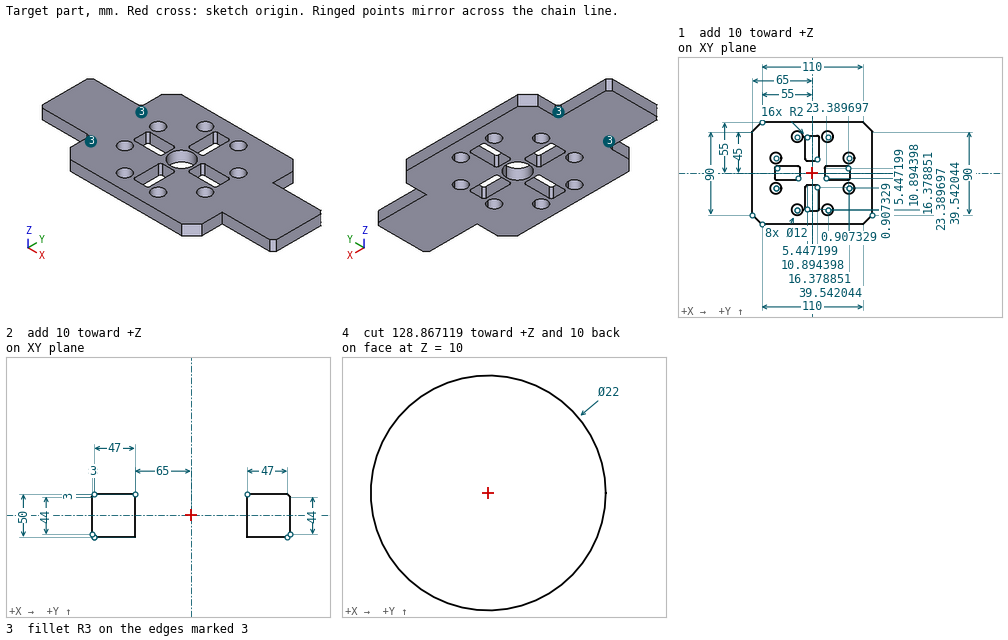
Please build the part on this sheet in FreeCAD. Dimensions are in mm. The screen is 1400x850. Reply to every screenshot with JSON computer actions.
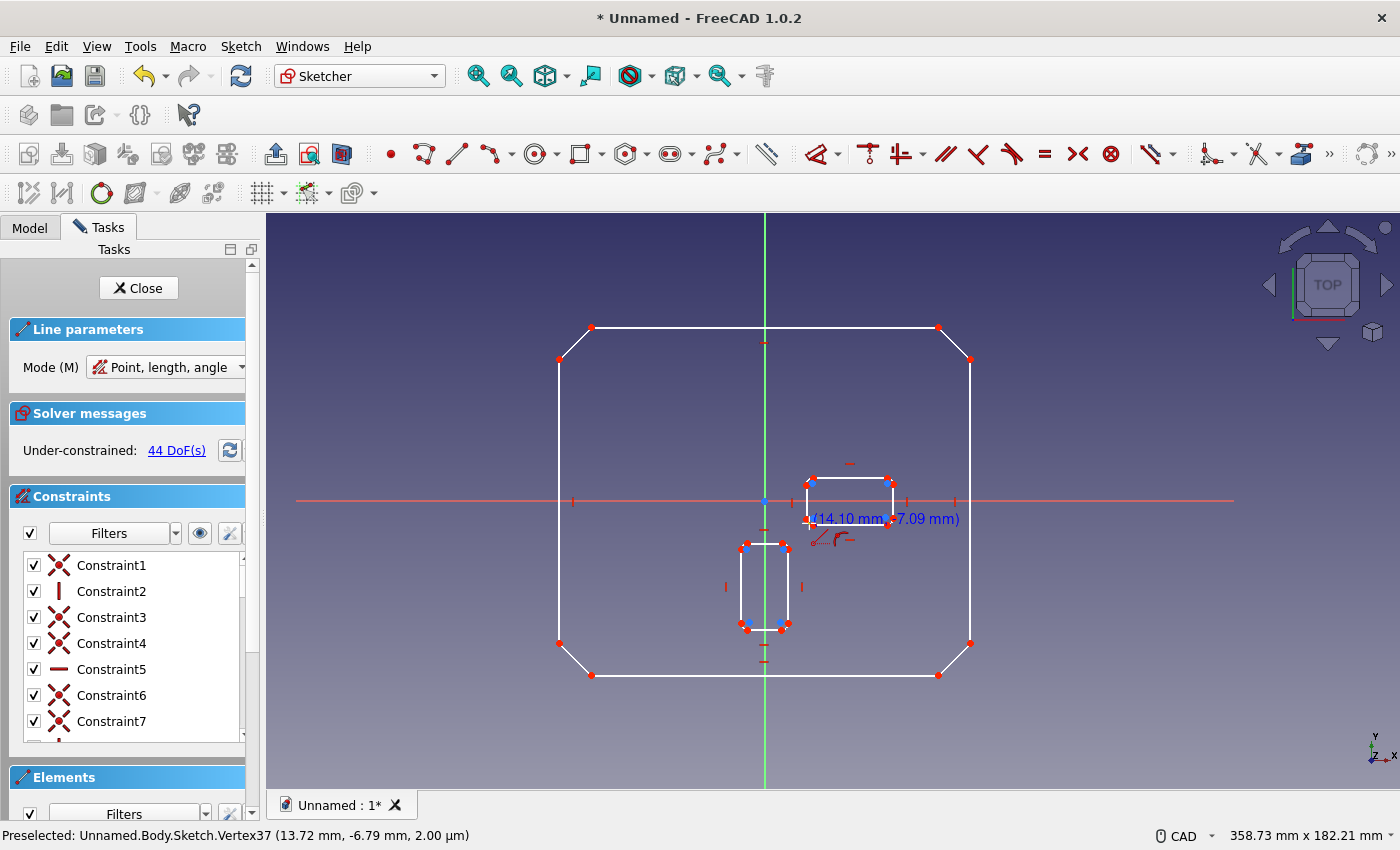
{"action": "left_click", "coordinate": [723, 484]}
{"action": "left_click", "coordinate": [723, 518]}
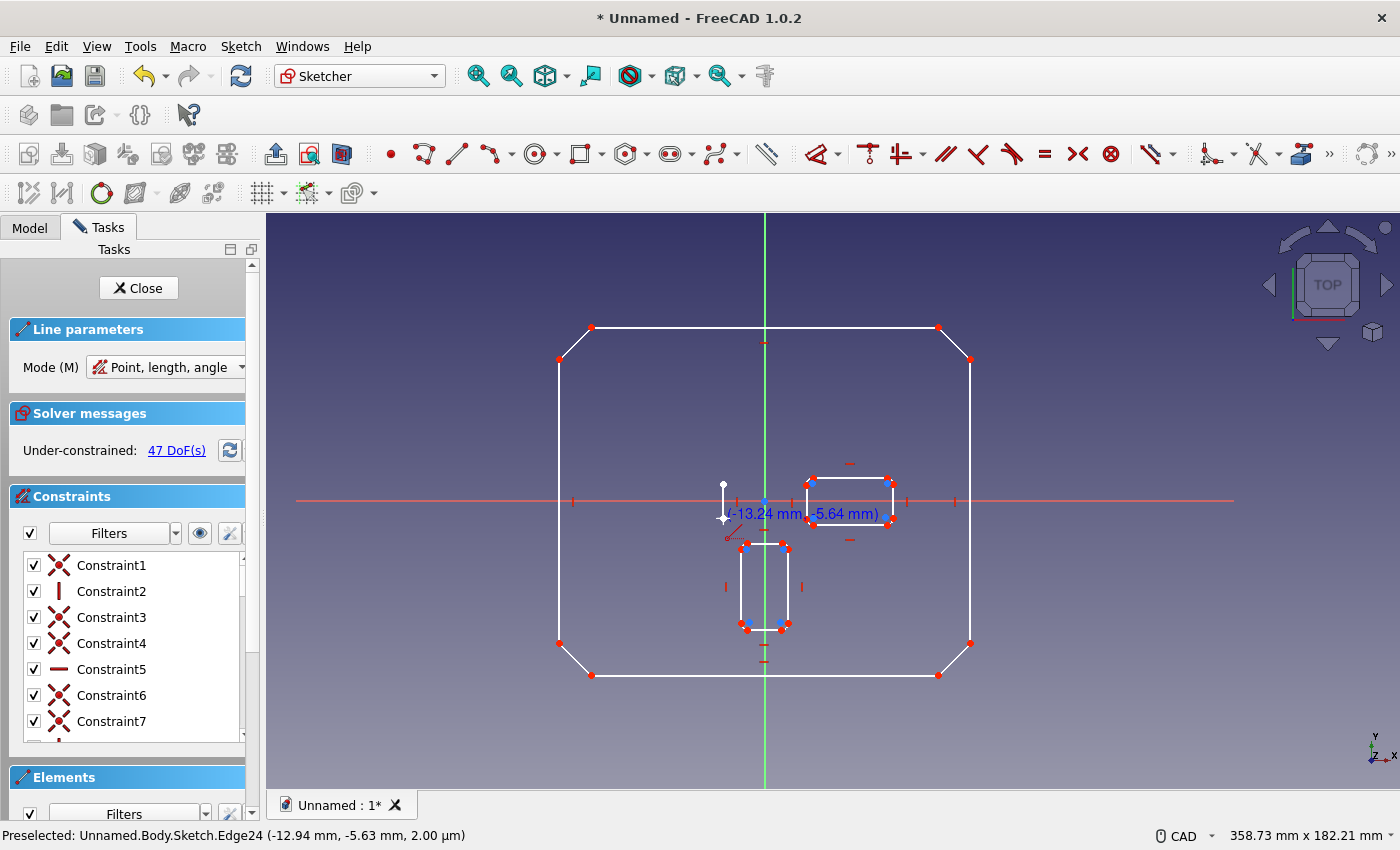
{"action": "scroll", "coordinate": [717, 525], "scroll_direction": "up", "scroll_amount": 3}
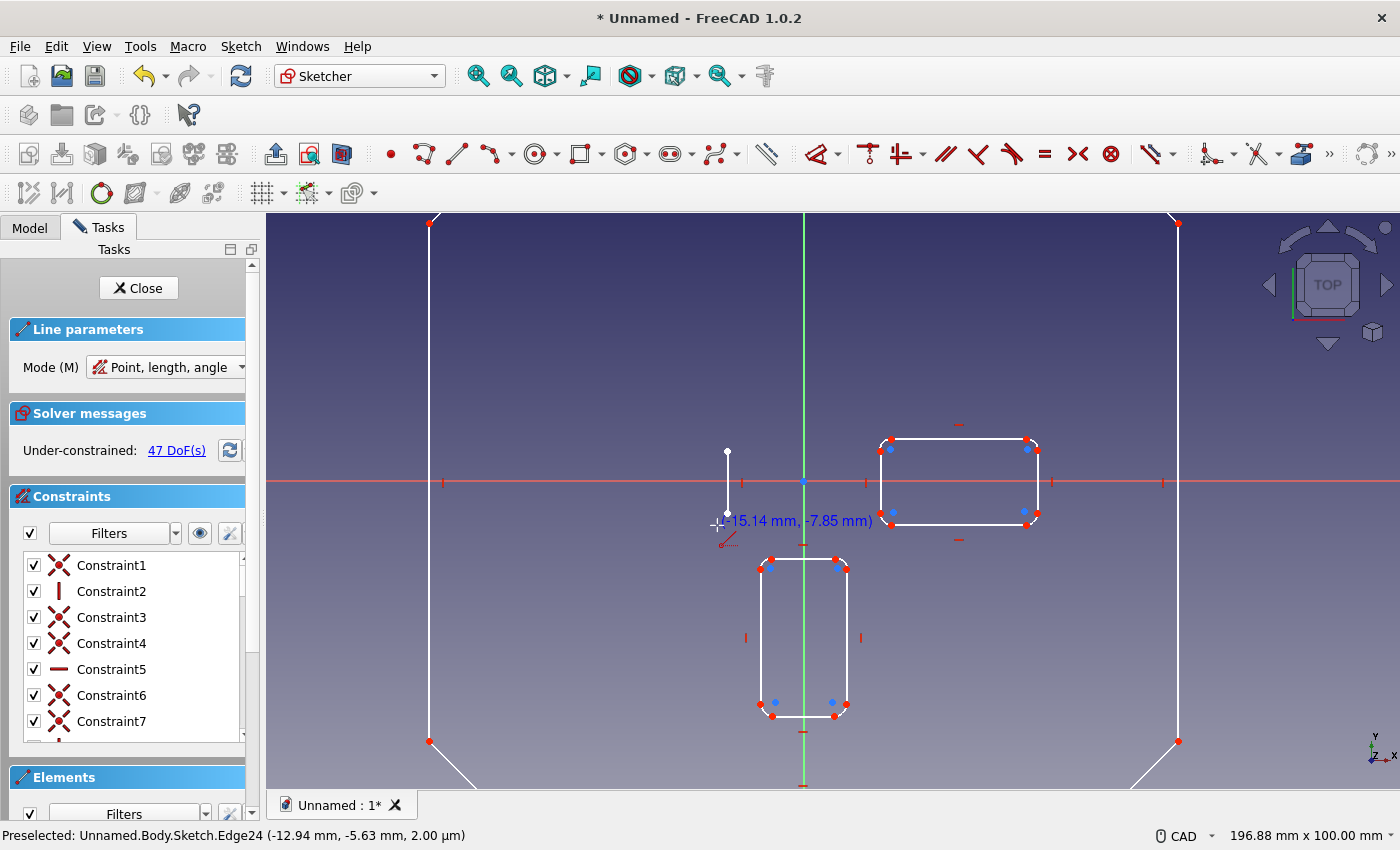
{"action": "left_click", "coordinate": [716, 524]}
{"action": "left_click", "coordinate": [581, 524]}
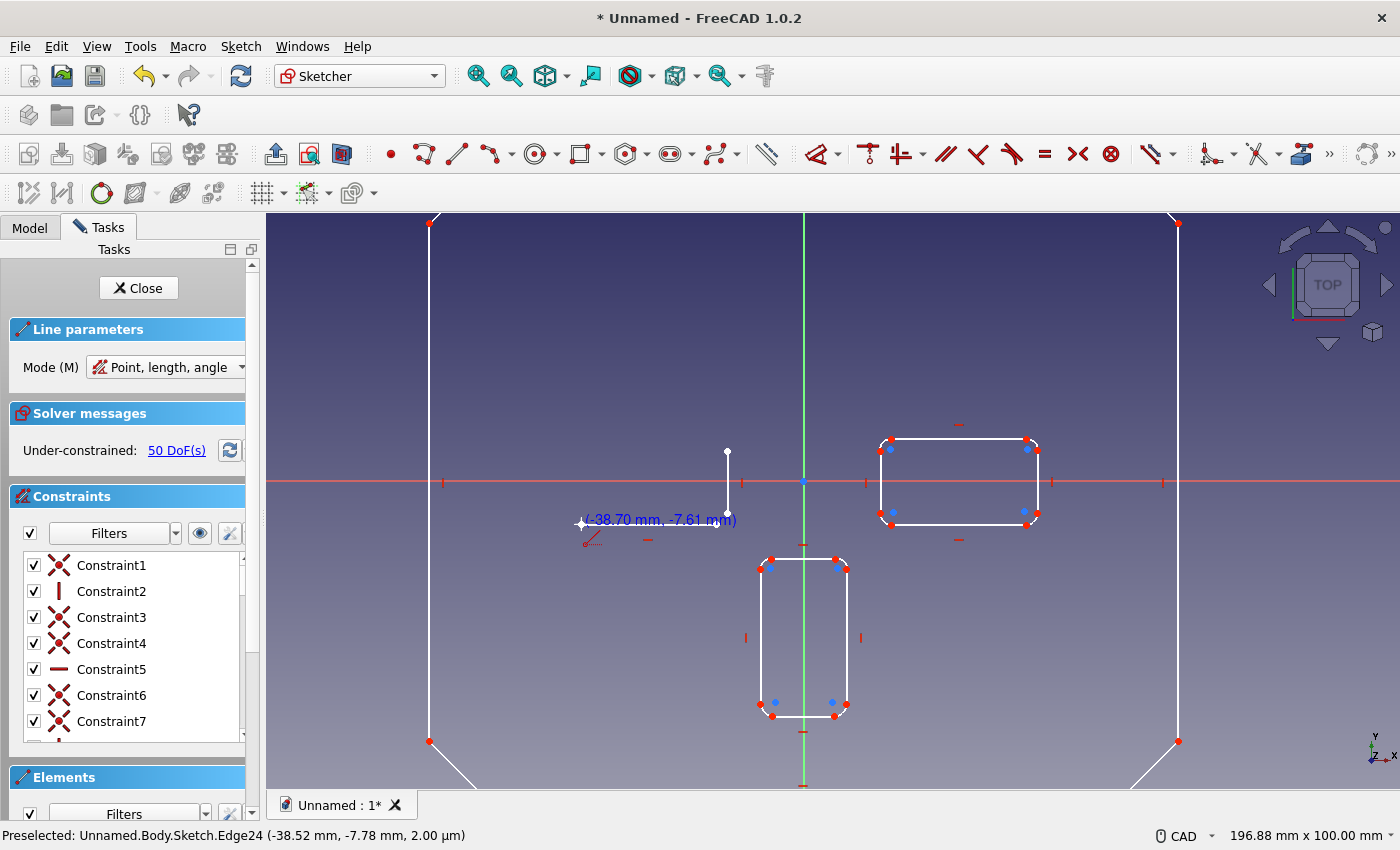
{"action": "left_click", "coordinate": [570, 513]}
{"action": "left_click", "coordinate": [570, 450]}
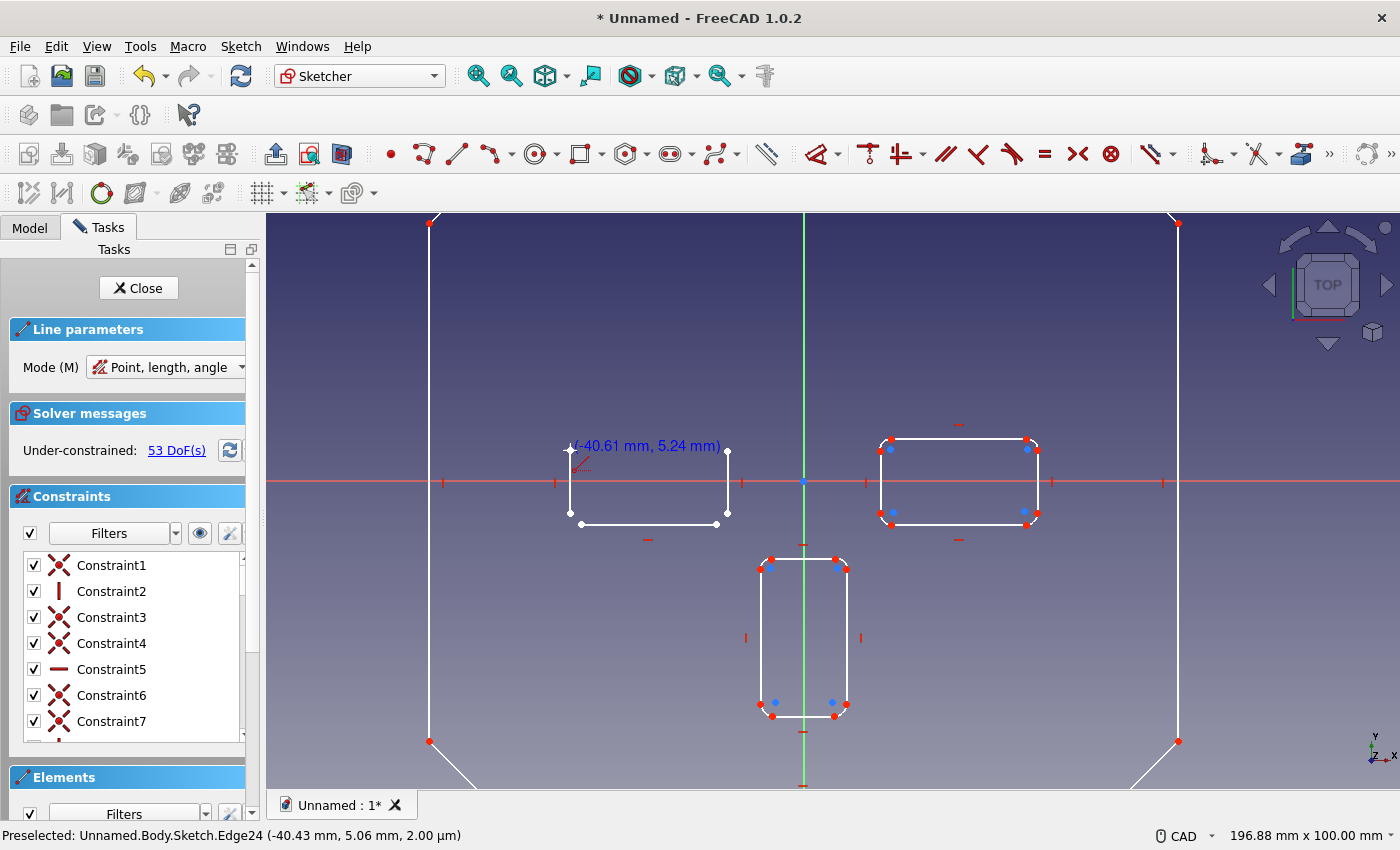
{"action": "left_click", "coordinate": [581, 438]}
{"action": "left_click", "coordinate": [716, 438]}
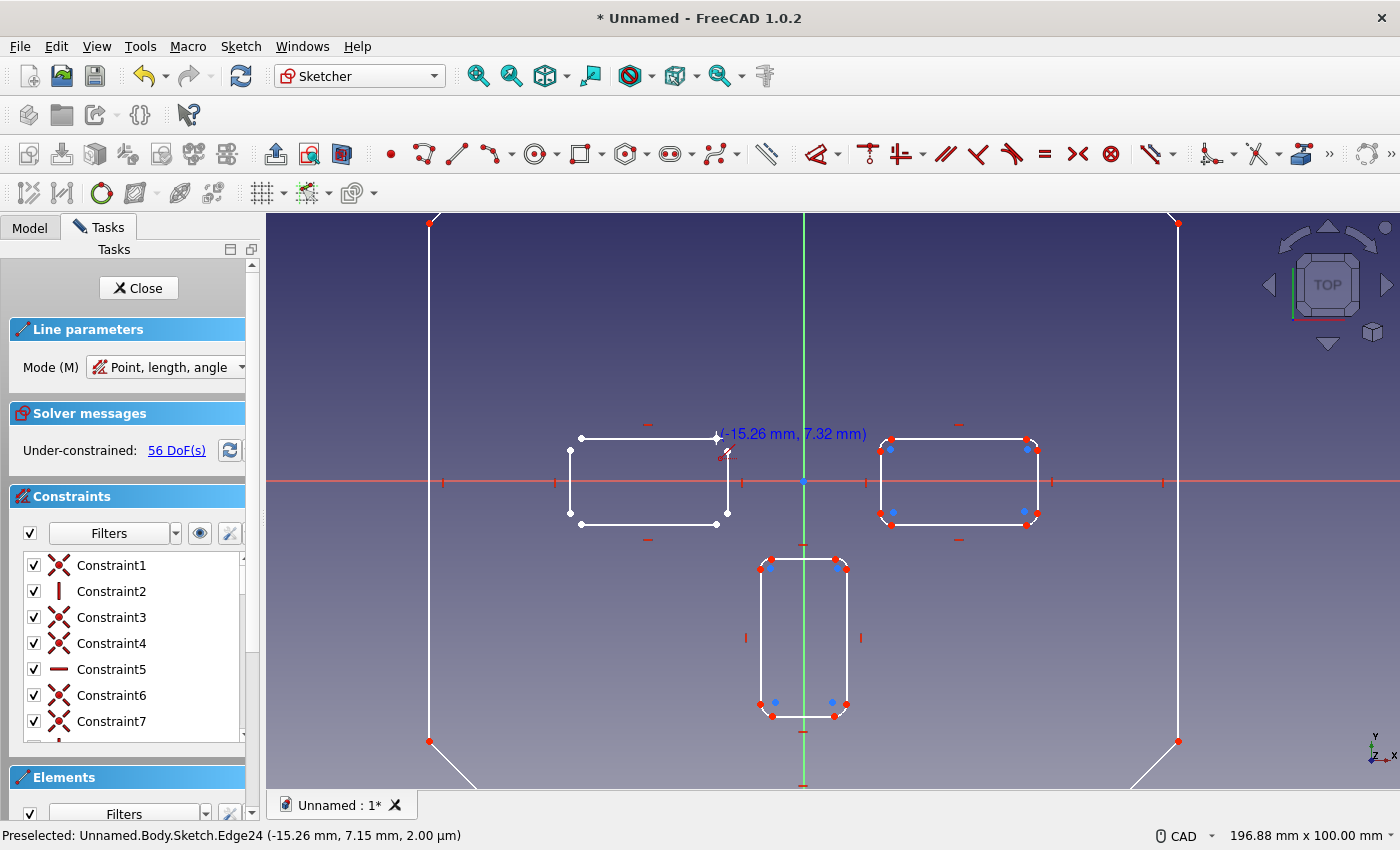
{"action": "left_click", "coordinate": [490, 154]}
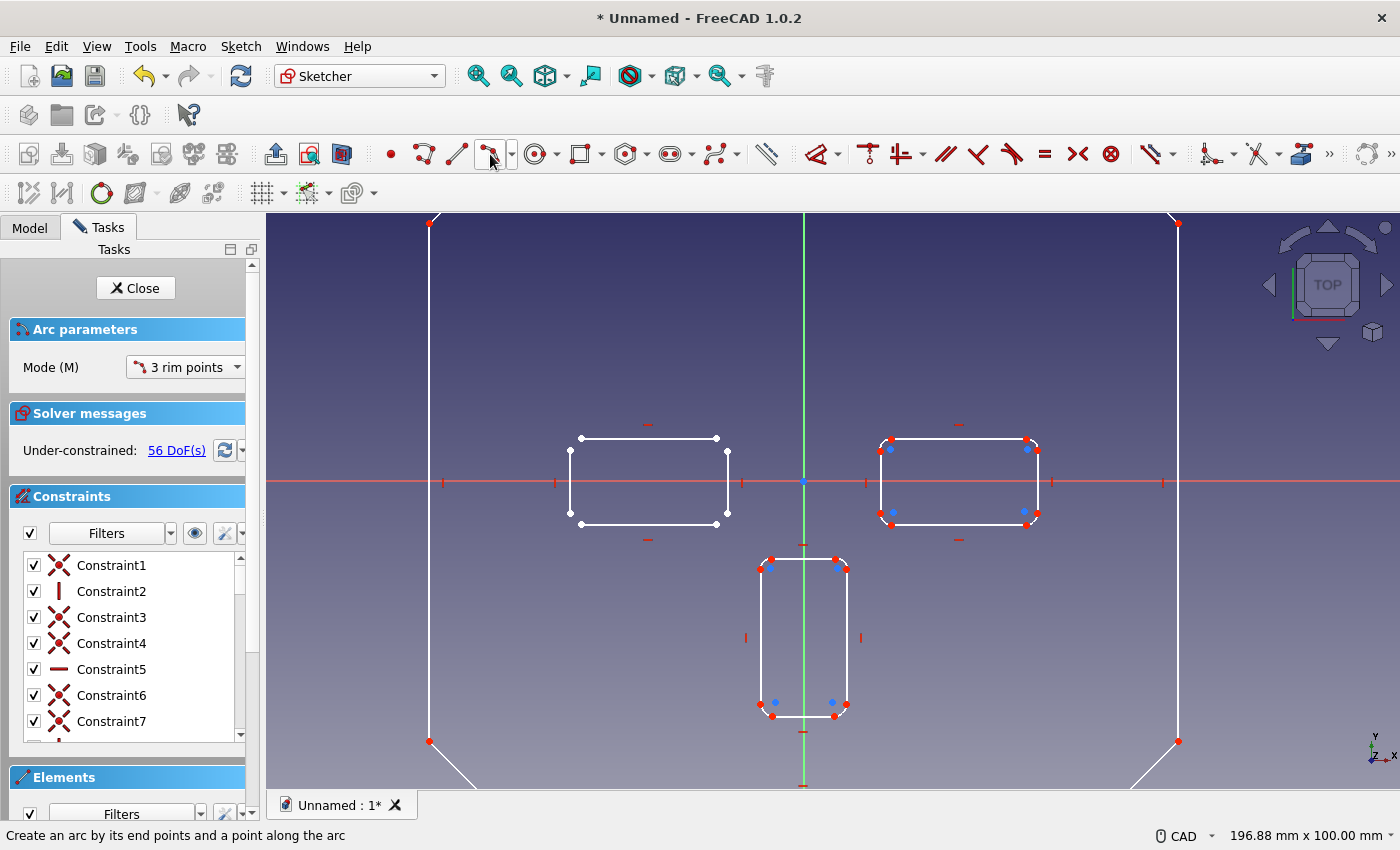
{"action": "left_click", "coordinate": [728, 514]}
{"action": "left_click", "coordinate": [716, 525]}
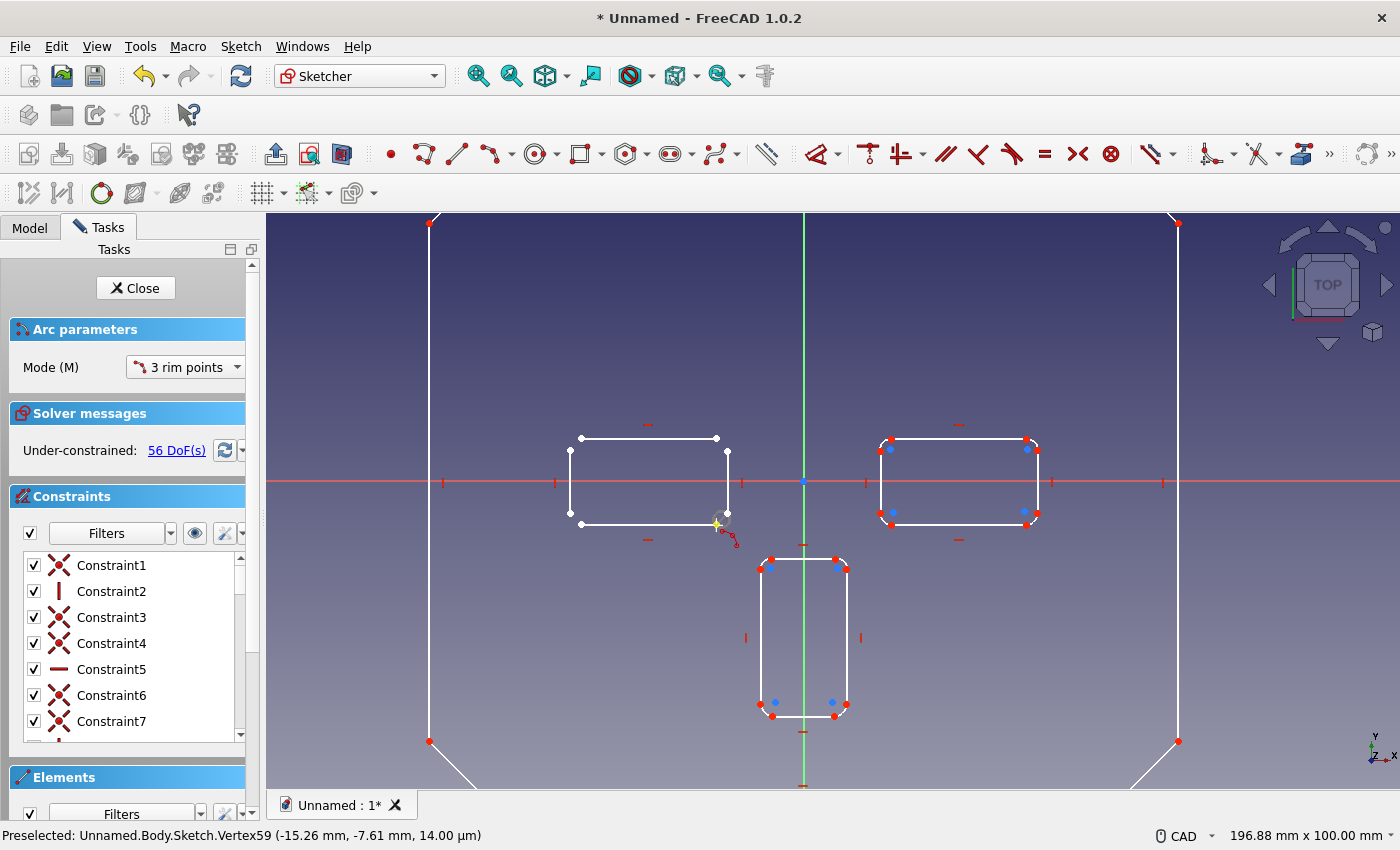
{"action": "scroll", "coordinate": [724, 521], "scroll_direction": "up", "scroll_amount": 8}